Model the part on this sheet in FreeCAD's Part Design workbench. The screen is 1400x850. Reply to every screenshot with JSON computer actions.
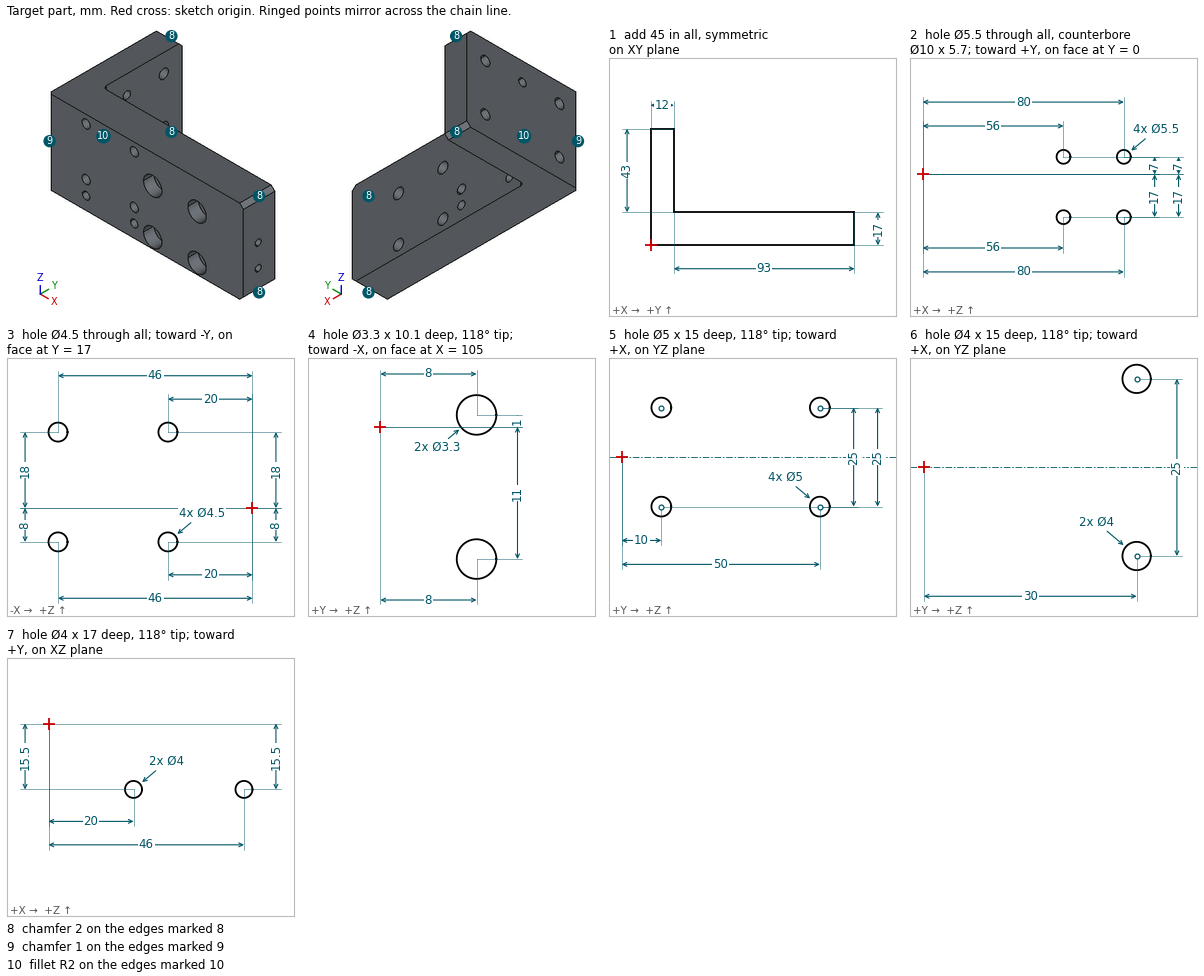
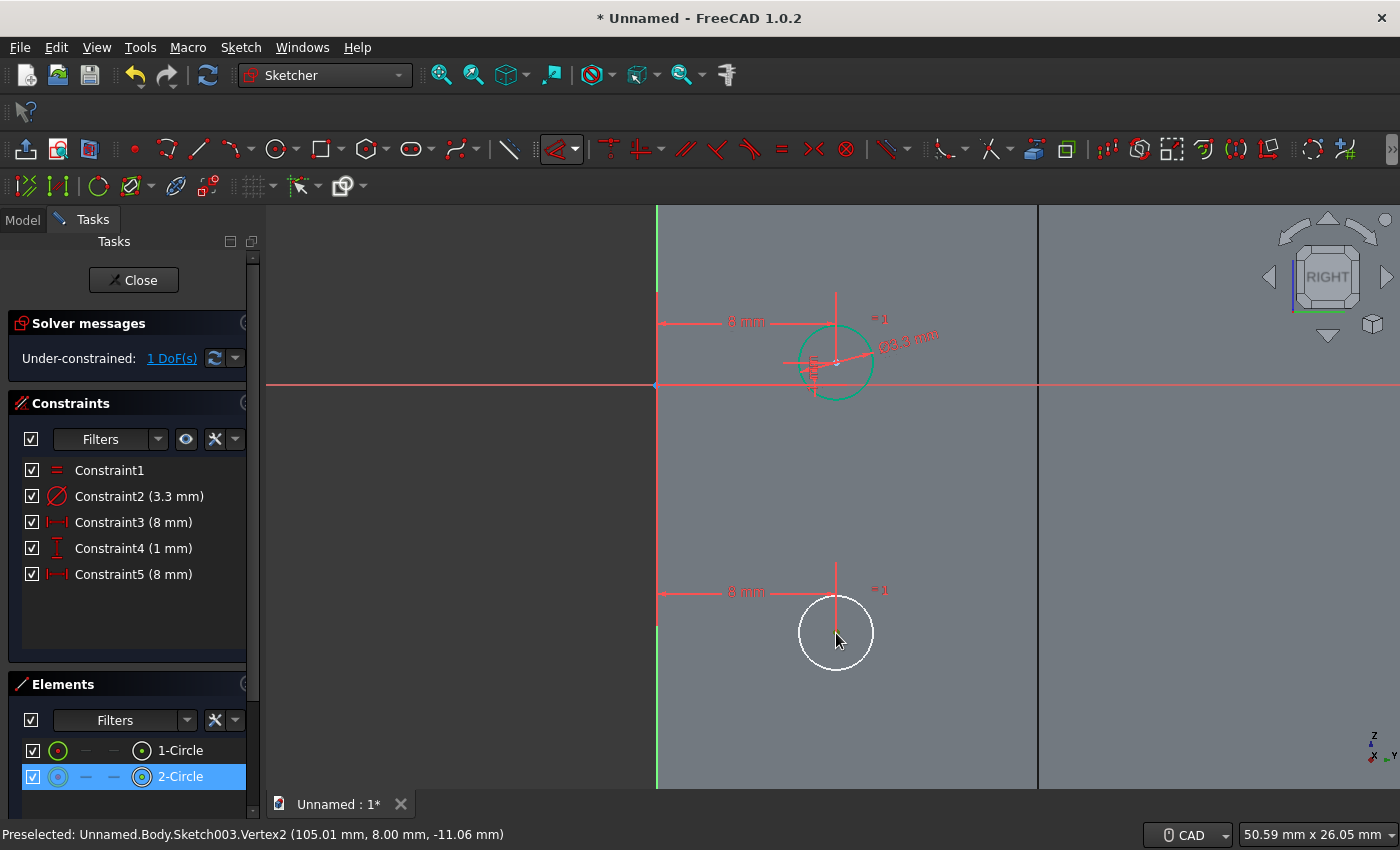
{"action": "key", "text": "i"}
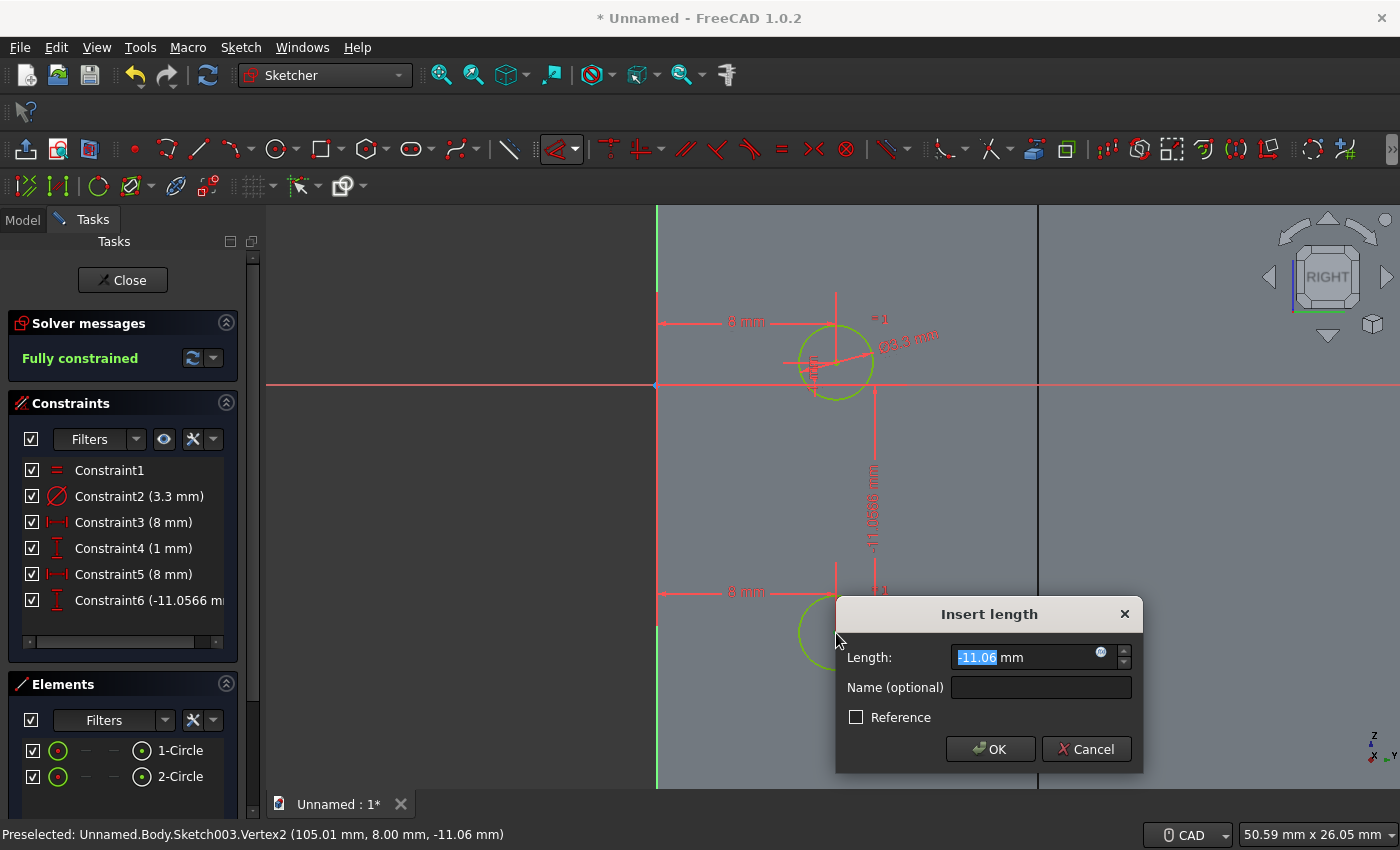
{"action": "type", "text": "-11"}
{"action": "key", "text": "Return"}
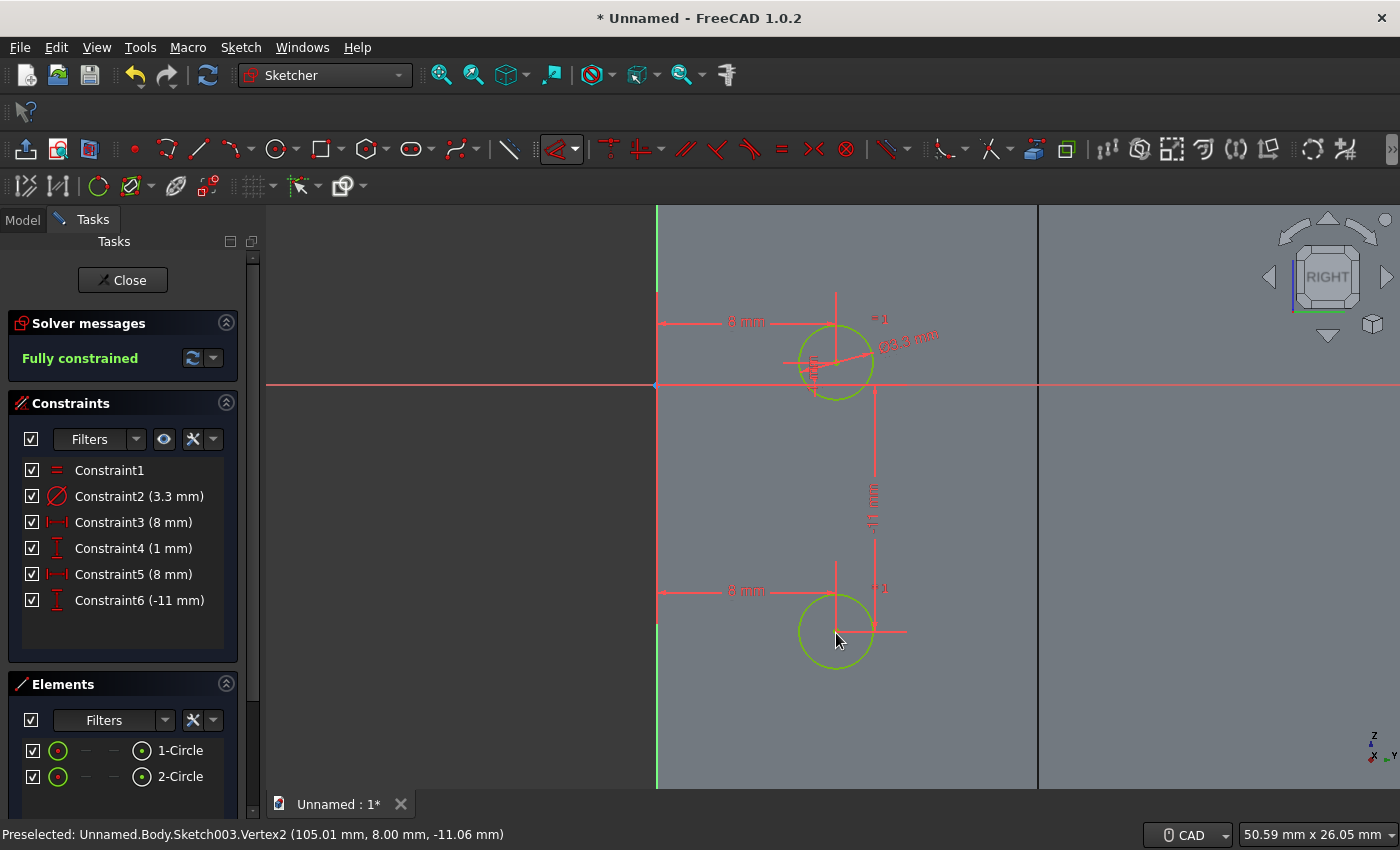
{"action": "left_click", "coordinate": [123, 280]}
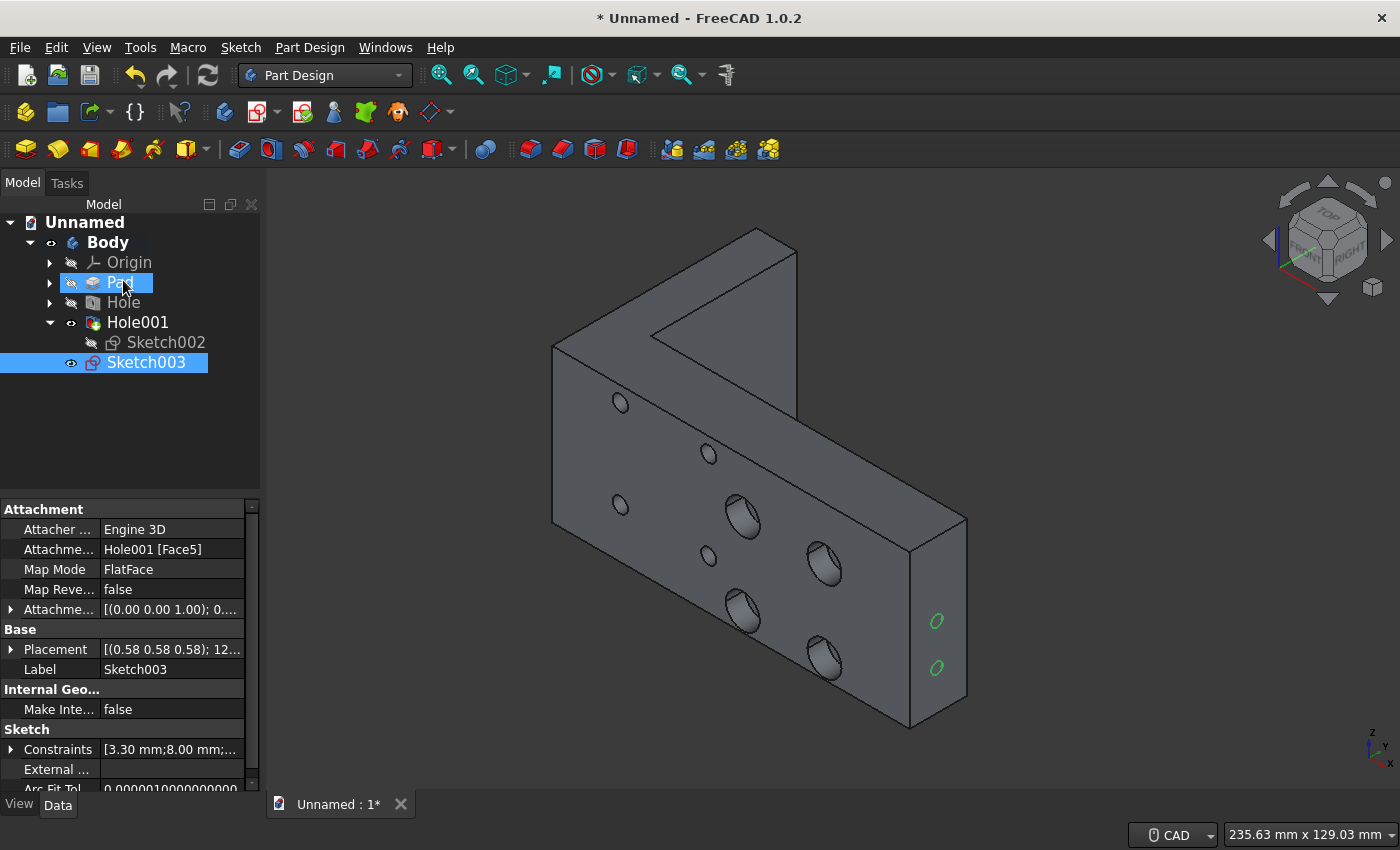
{"action": "left_click", "coordinate": [272, 150]}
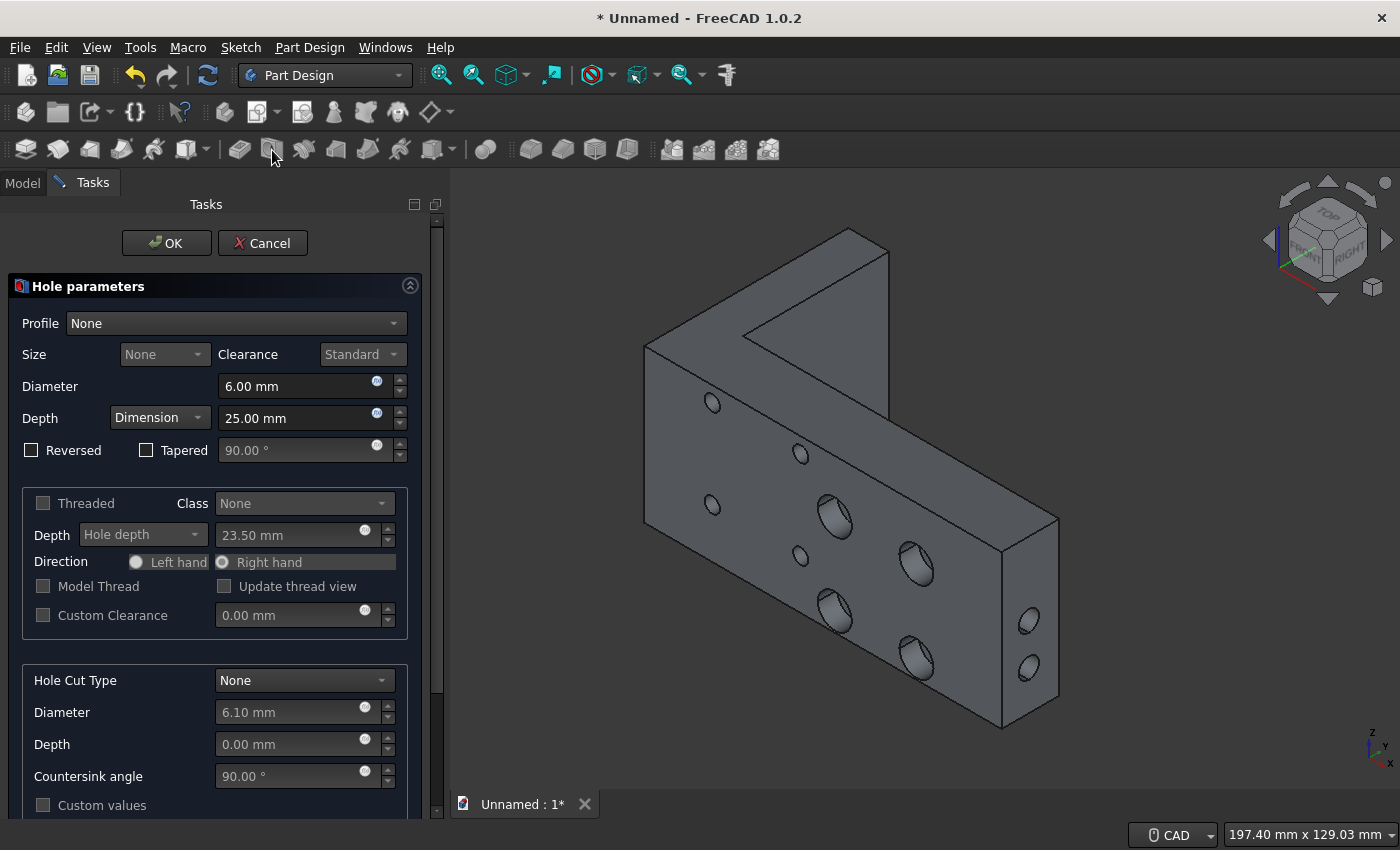
{"action": "triple_click", "coordinate": [305, 386]}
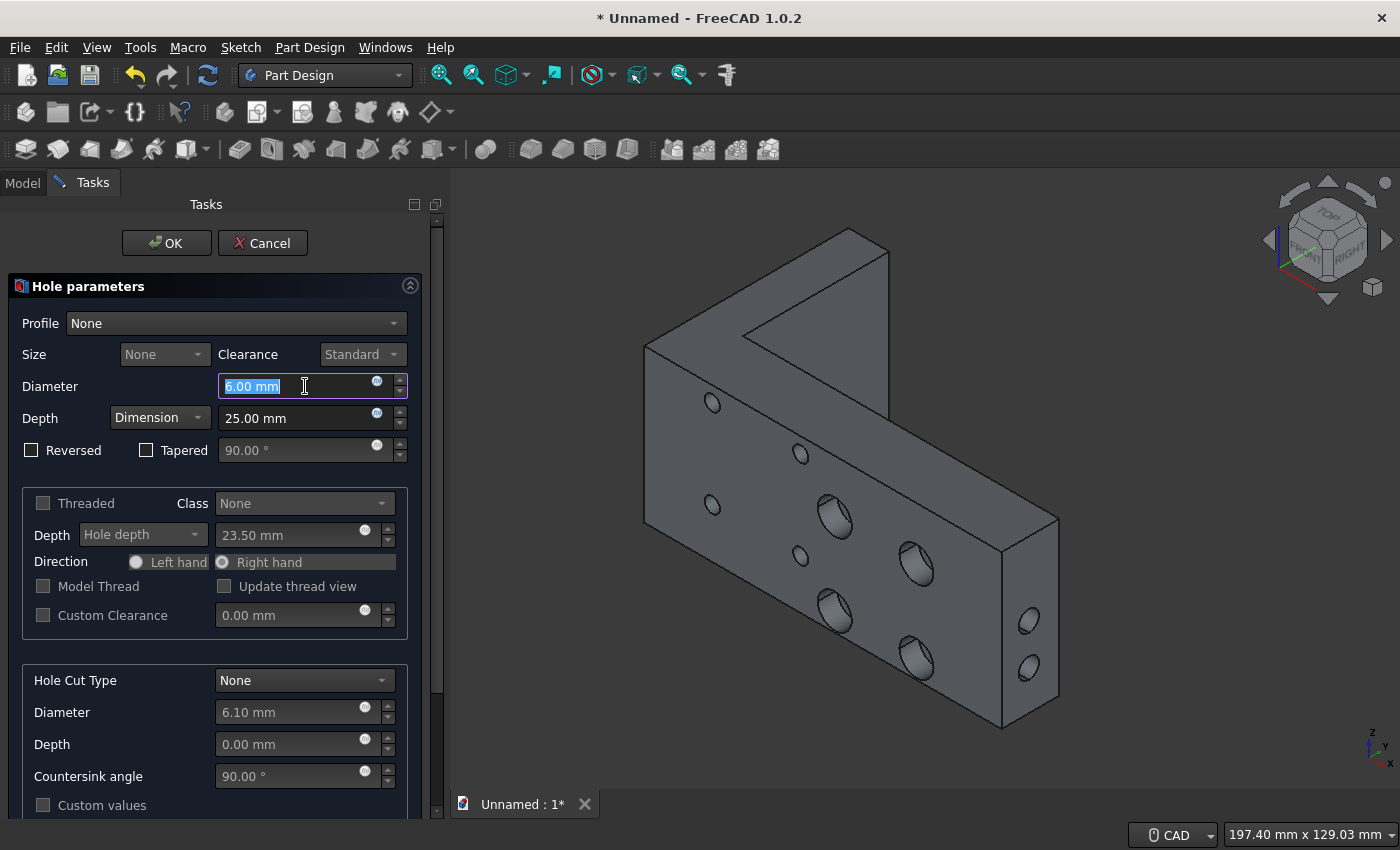
{"action": "type", "text": "3.3"}
{"action": "key", "text": "Tab"}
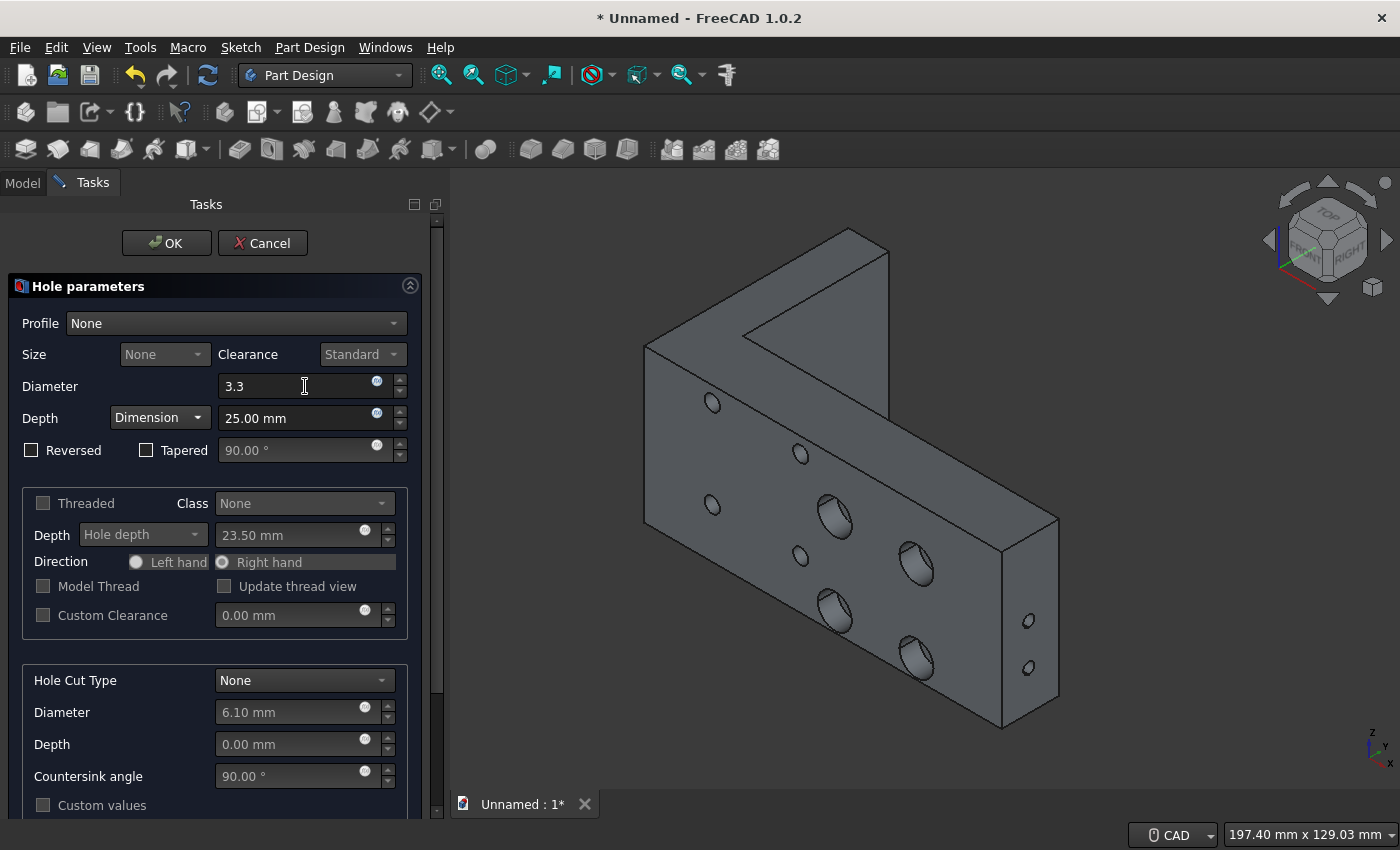
{"action": "triple_click", "coordinate": [305, 418]}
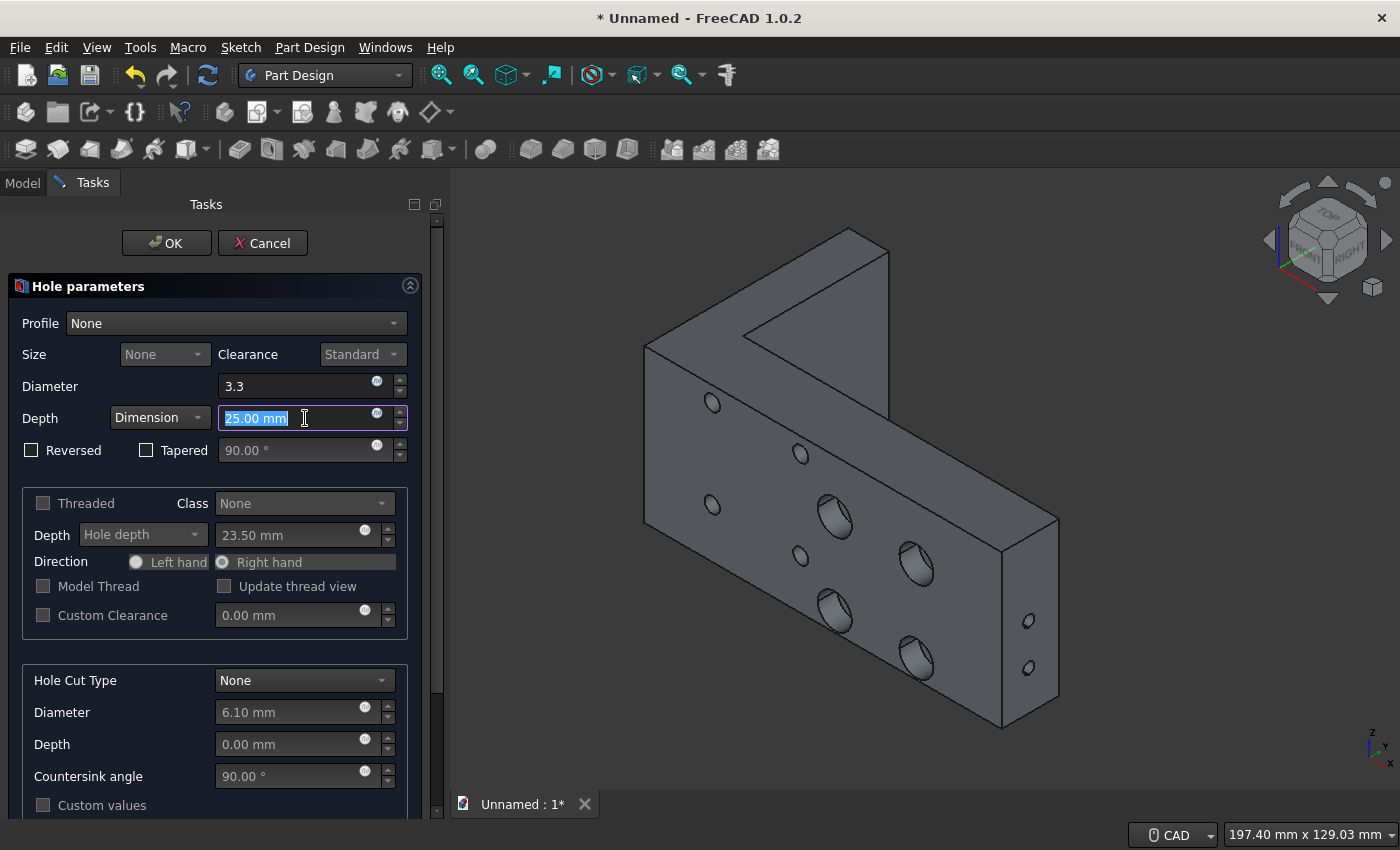
{"action": "type", "text": "10.1"}
{"action": "key", "text": "Tab"}